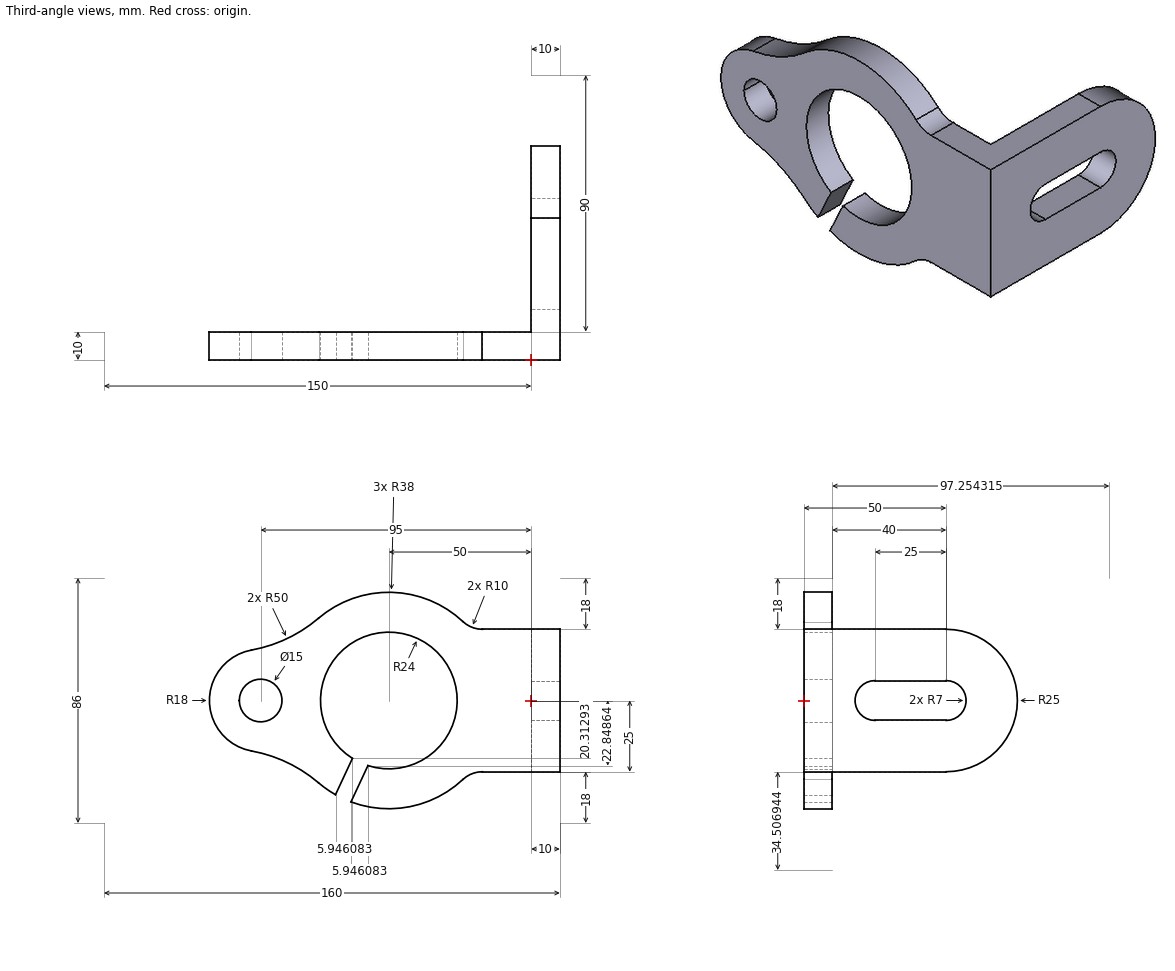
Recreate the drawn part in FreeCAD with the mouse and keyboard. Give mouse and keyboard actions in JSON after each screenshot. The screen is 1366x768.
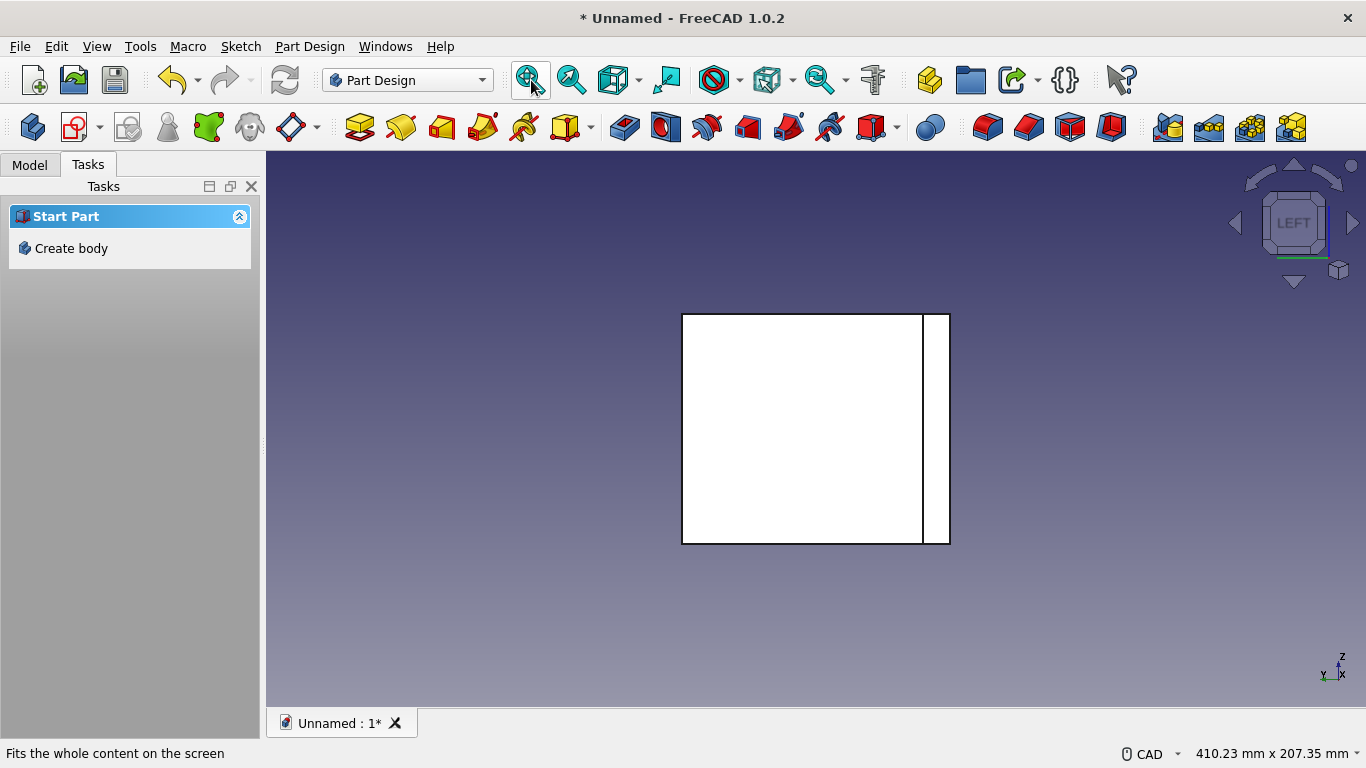
{"action": "left_click", "coordinate": [531, 80]}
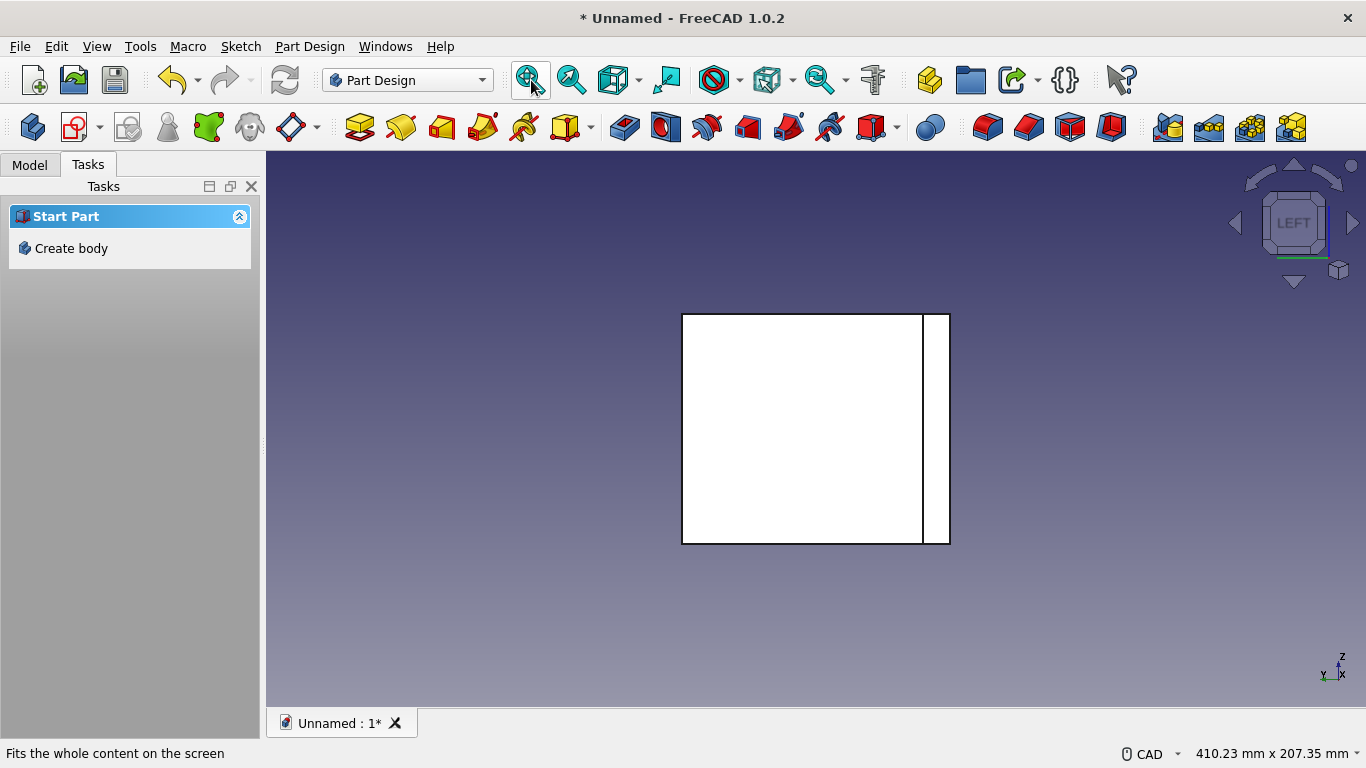
{"action": "left_click", "coordinate": [803, 428]}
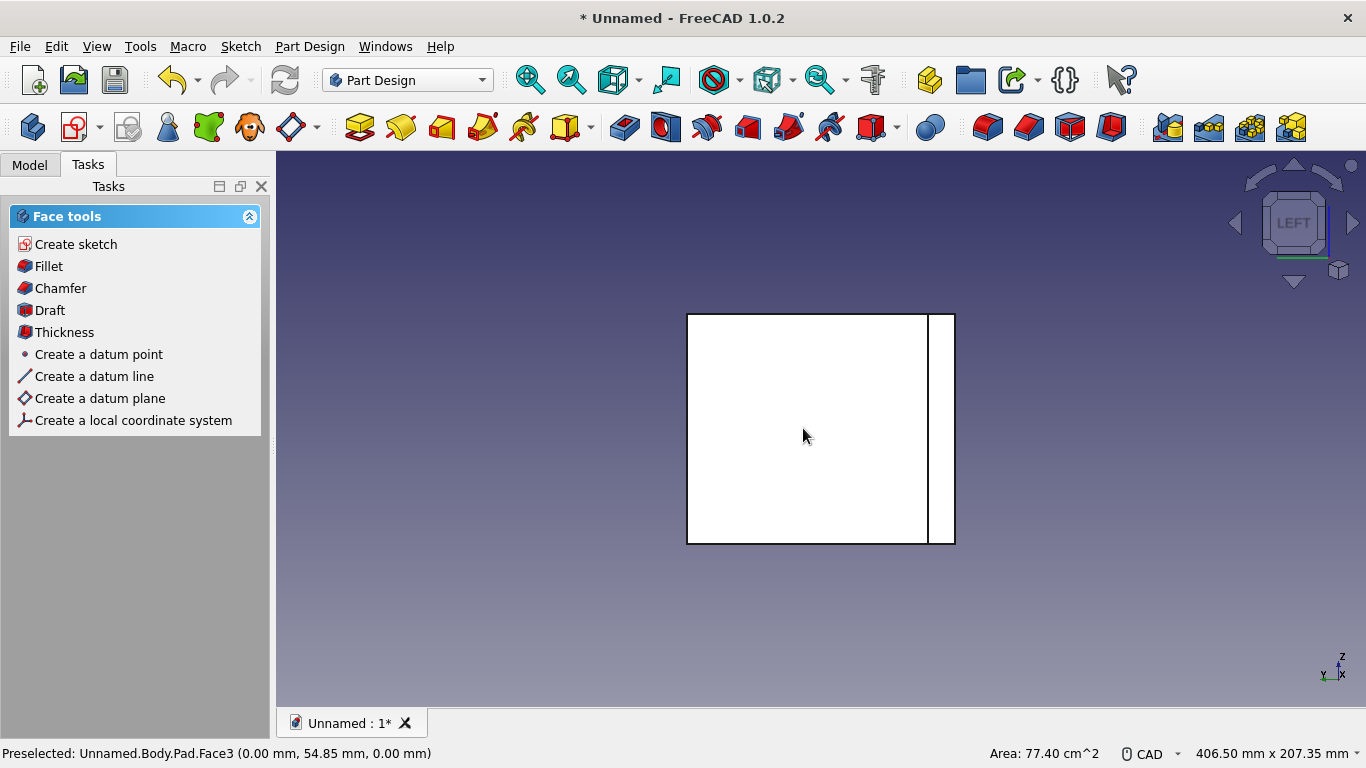
{"action": "left_click", "coordinate": [74, 128]}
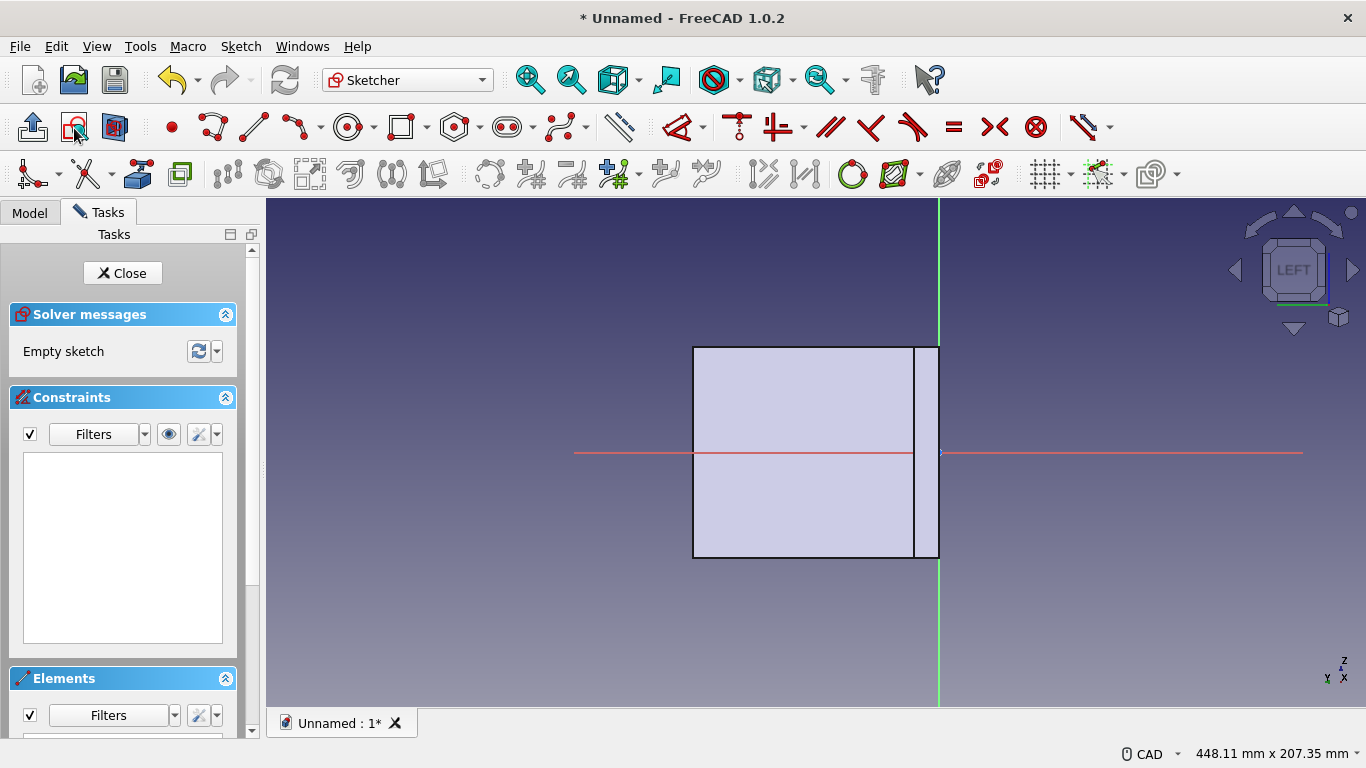
{"action": "key", "text": "g s"}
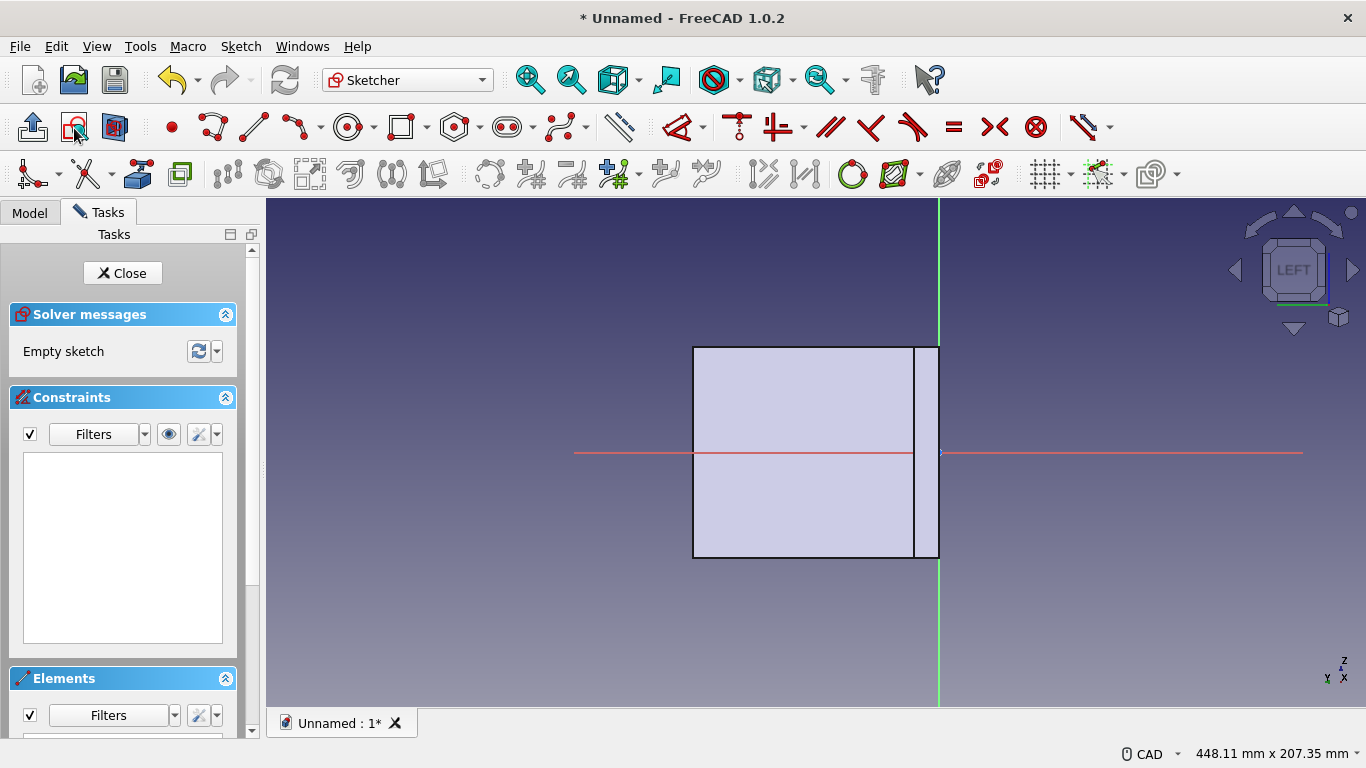
{"action": "scroll", "coordinate": [816, 452], "scroll_direction": "up", "scroll_amount": 2}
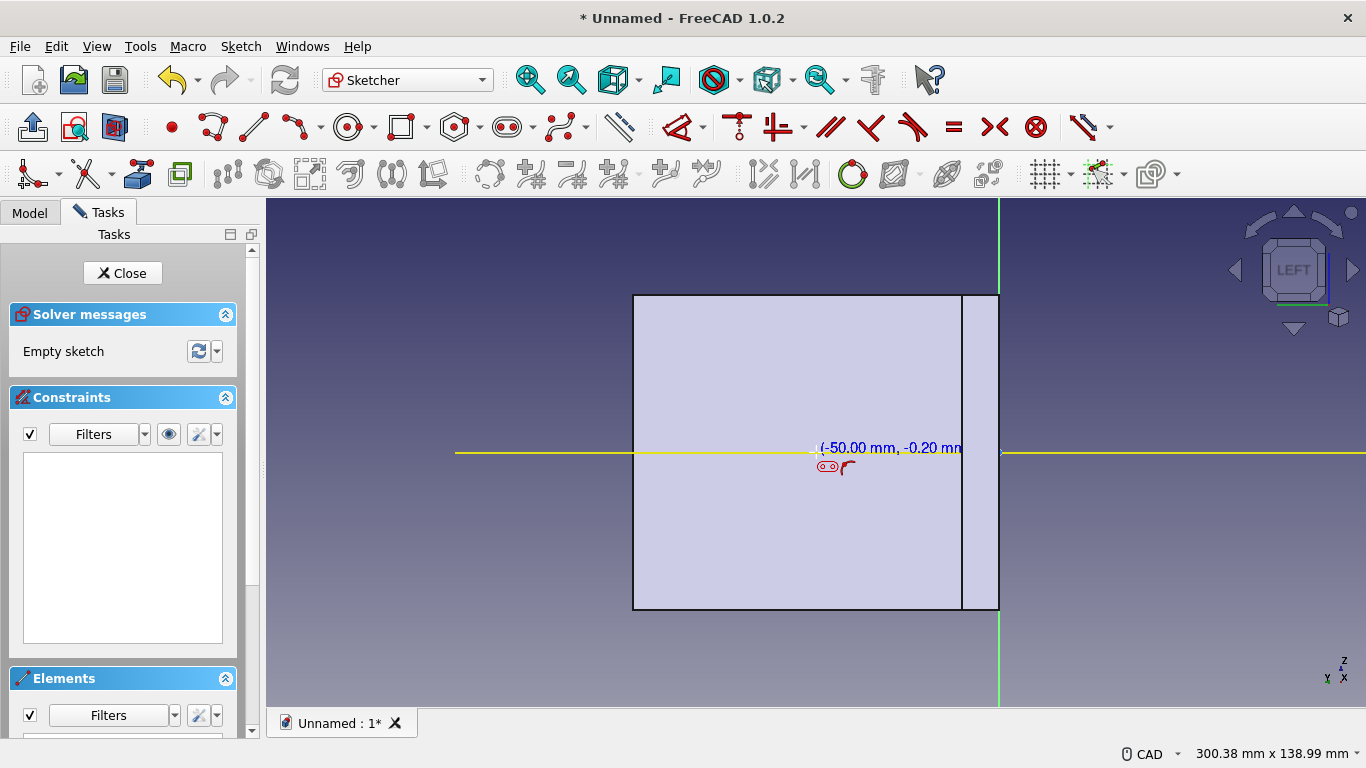
{"action": "left_click", "coordinate": [816, 452]}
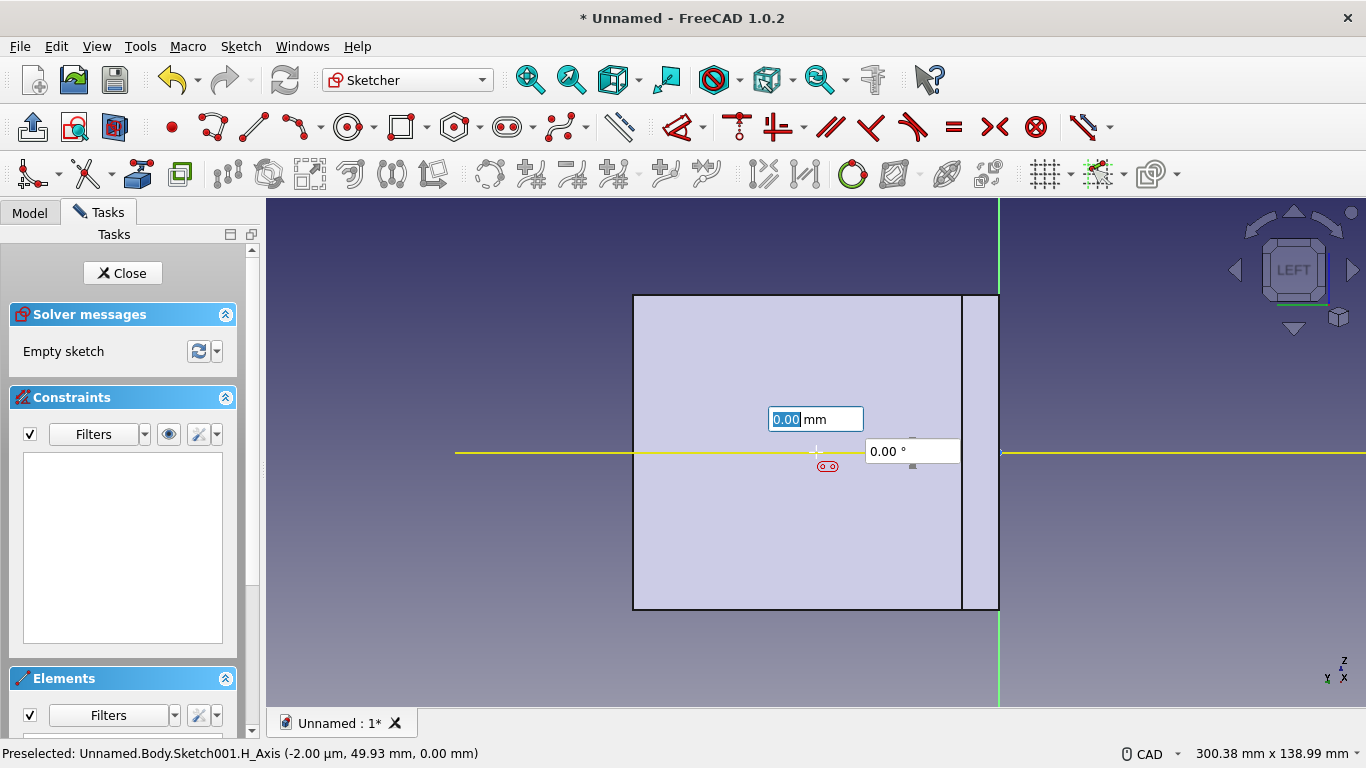
{"action": "left_click", "coordinate": [907, 462]}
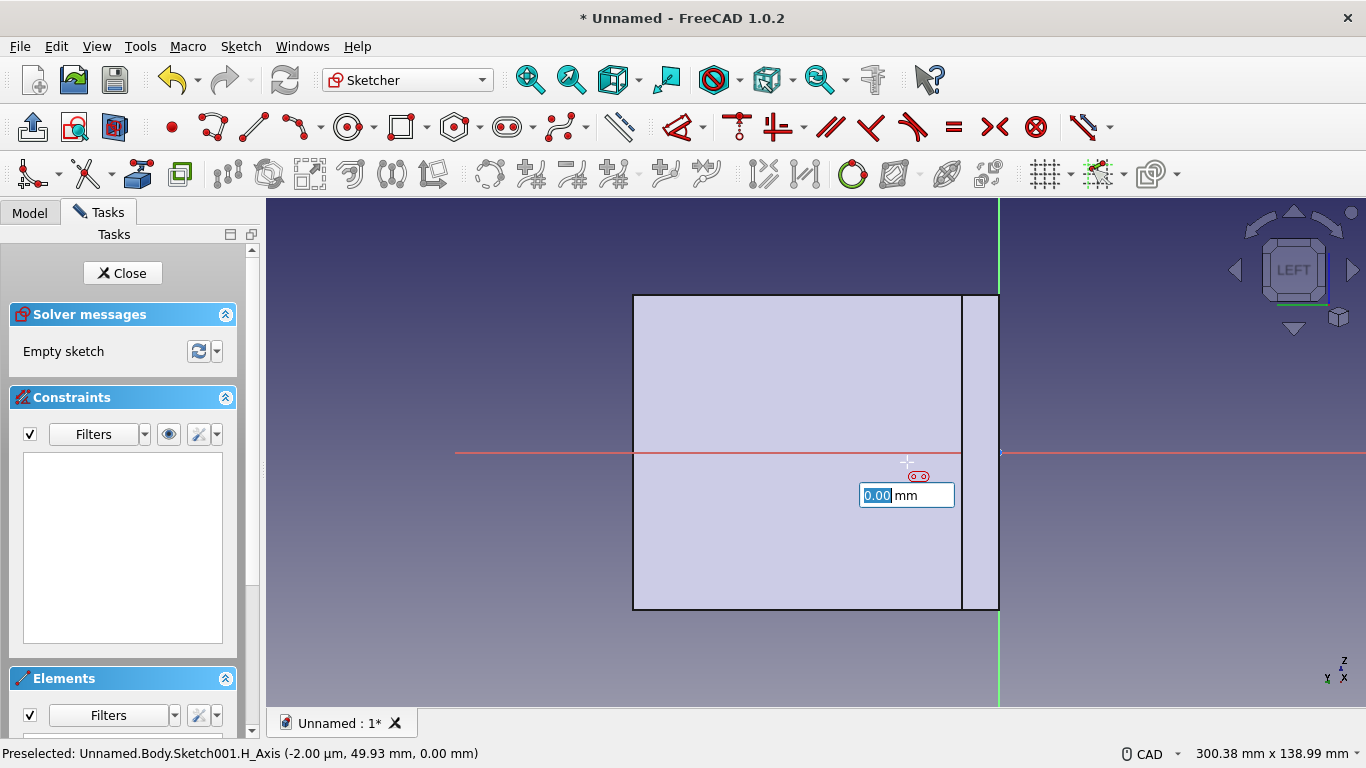
{"action": "left_click", "coordinate": [862, 427]}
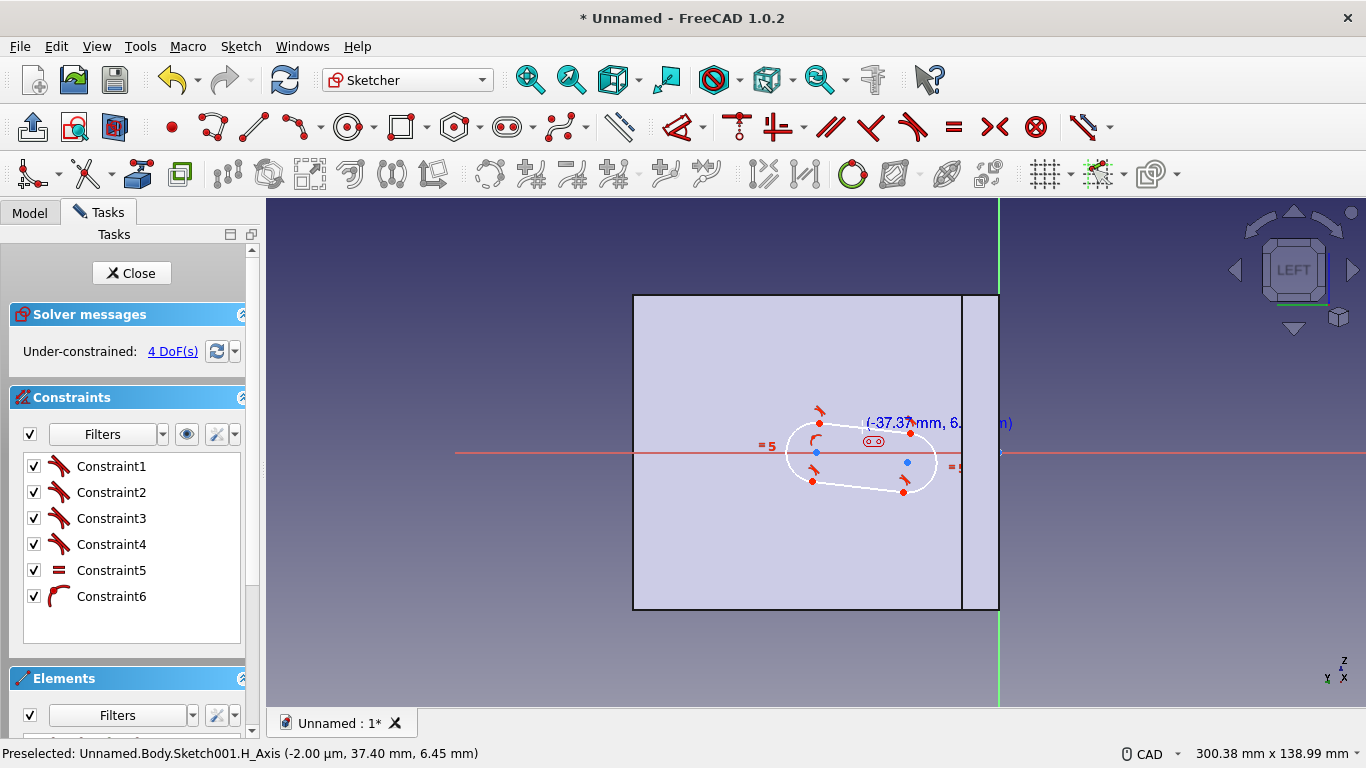
{"action": "key", "text": "g m"}